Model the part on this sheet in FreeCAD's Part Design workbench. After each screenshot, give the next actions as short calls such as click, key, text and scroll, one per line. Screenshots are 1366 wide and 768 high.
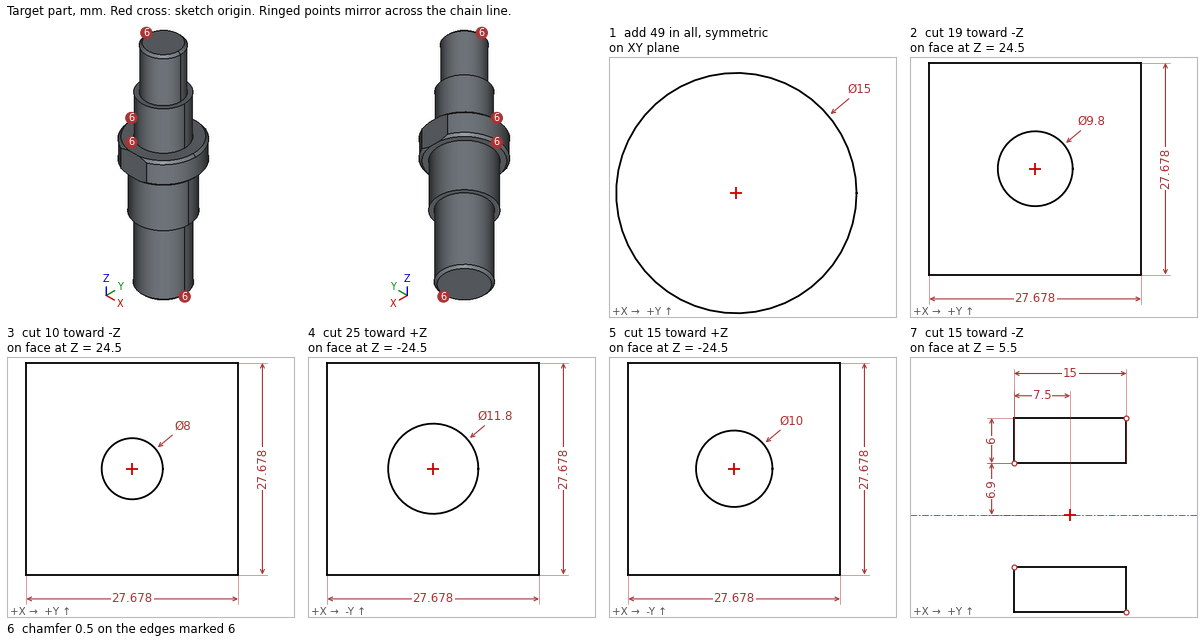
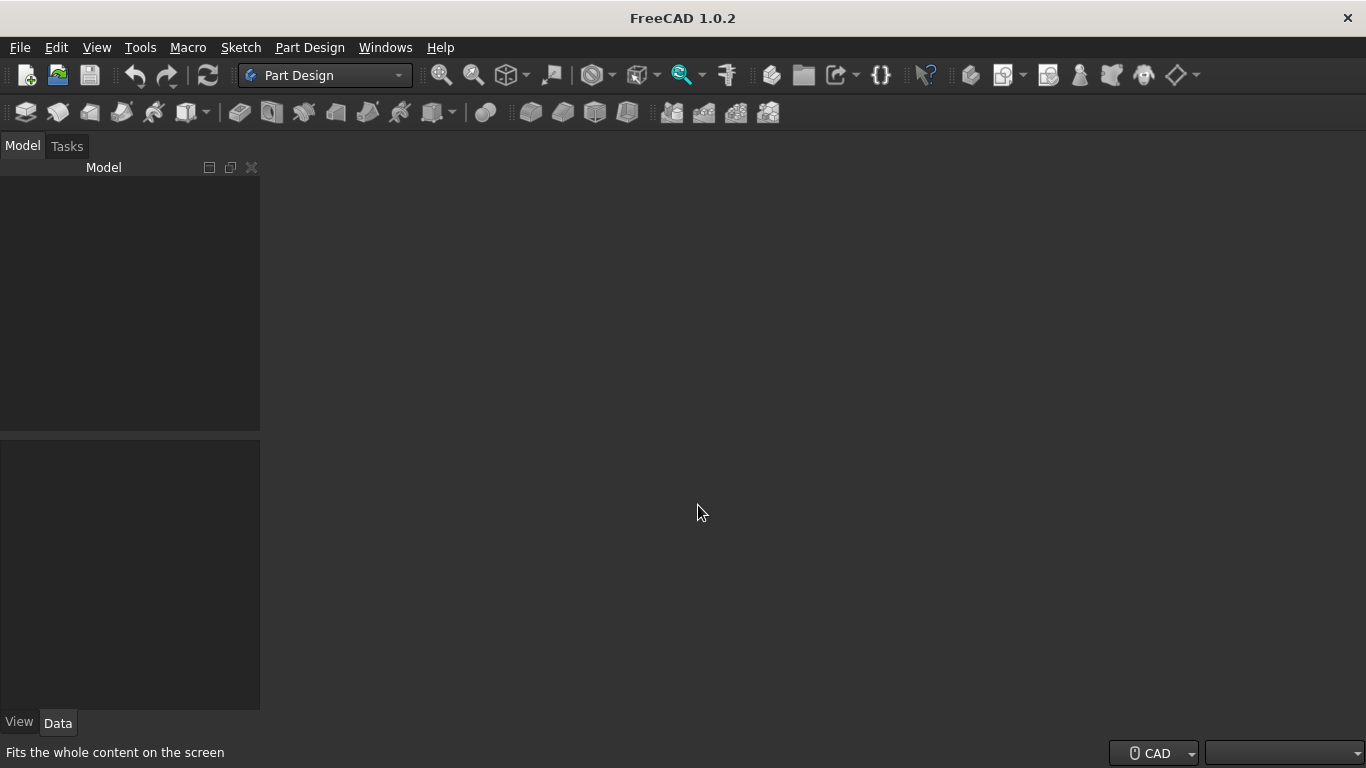
click(26, 76)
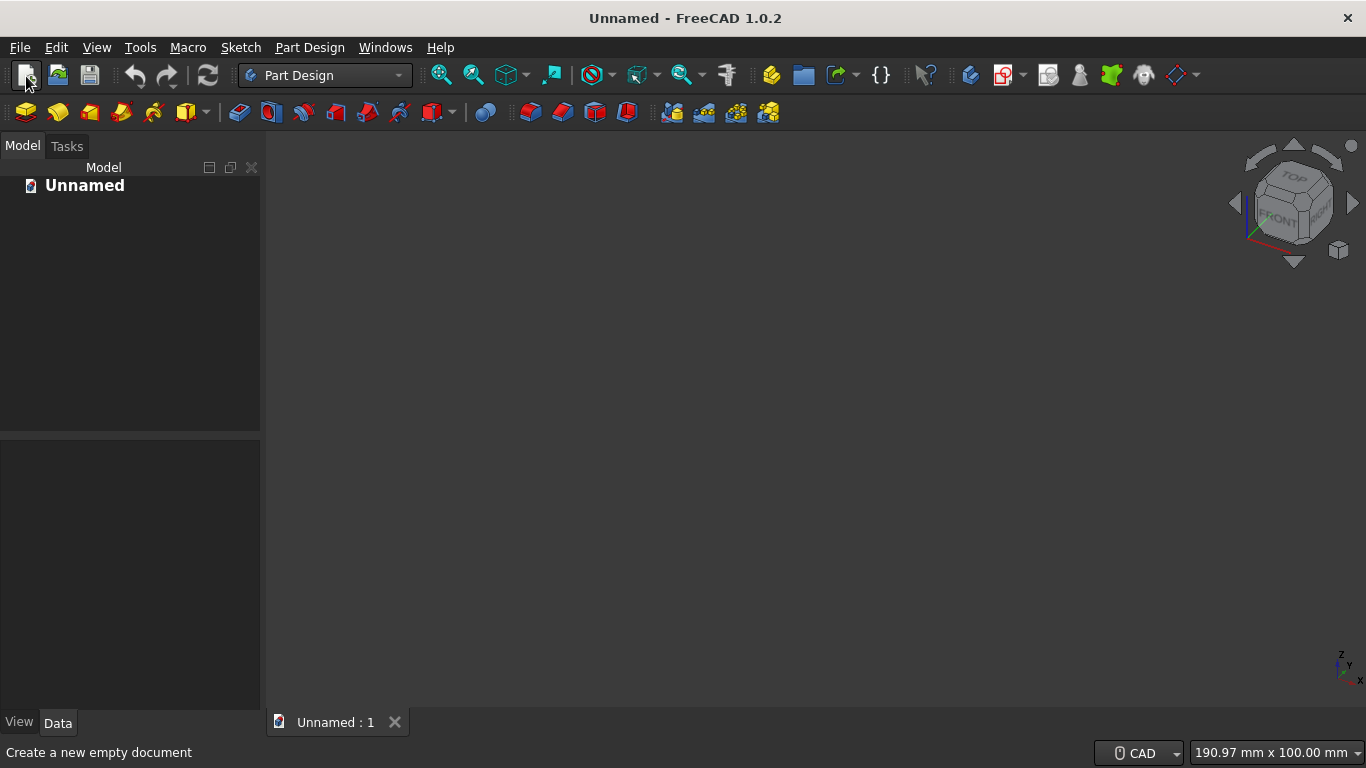
click(1004, 76)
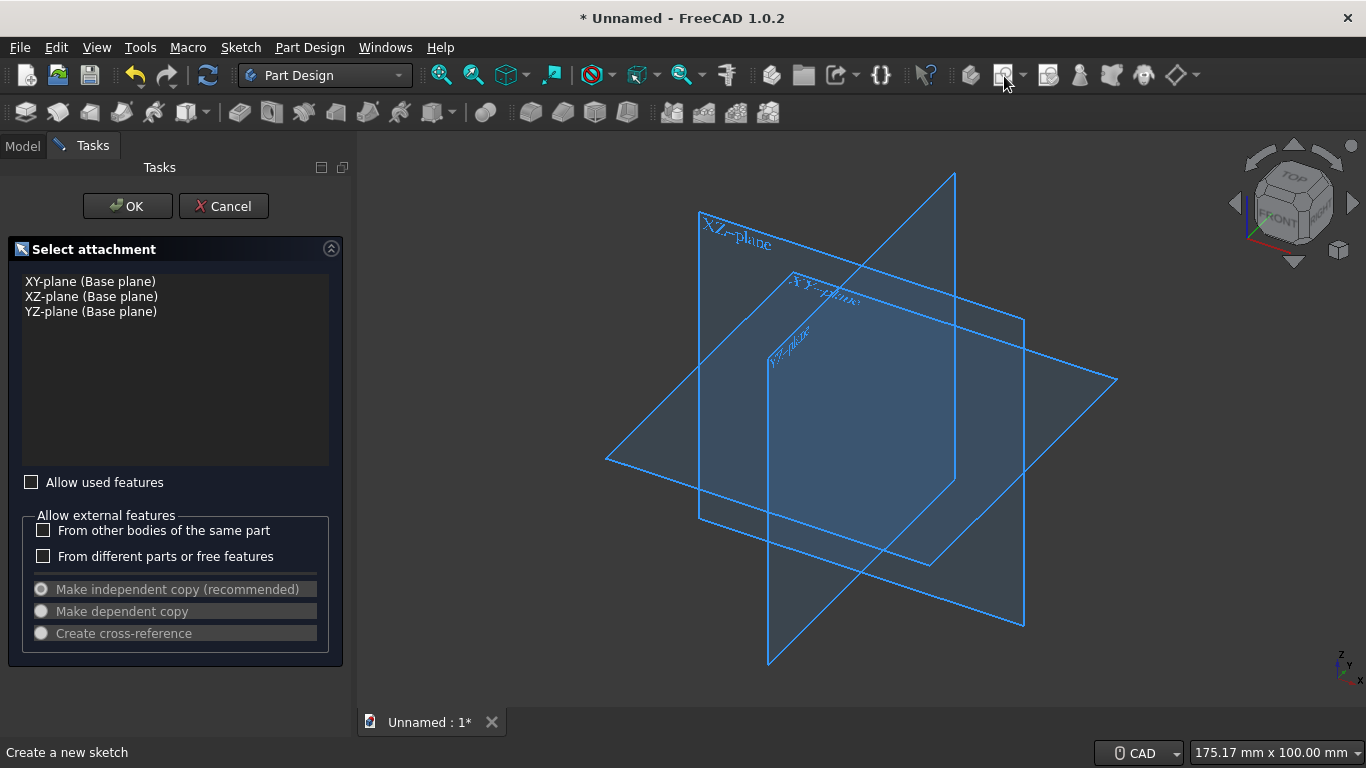
click(82, 282)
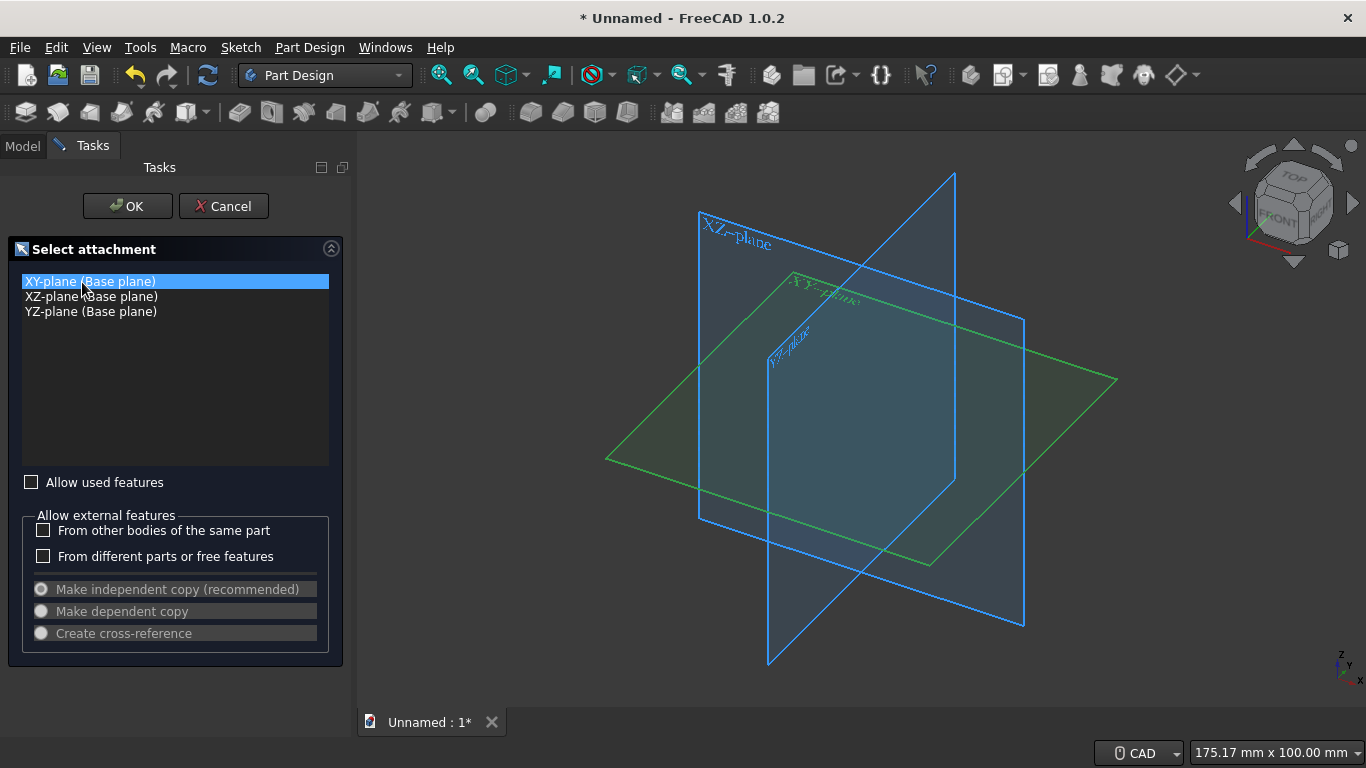
click(128, 206)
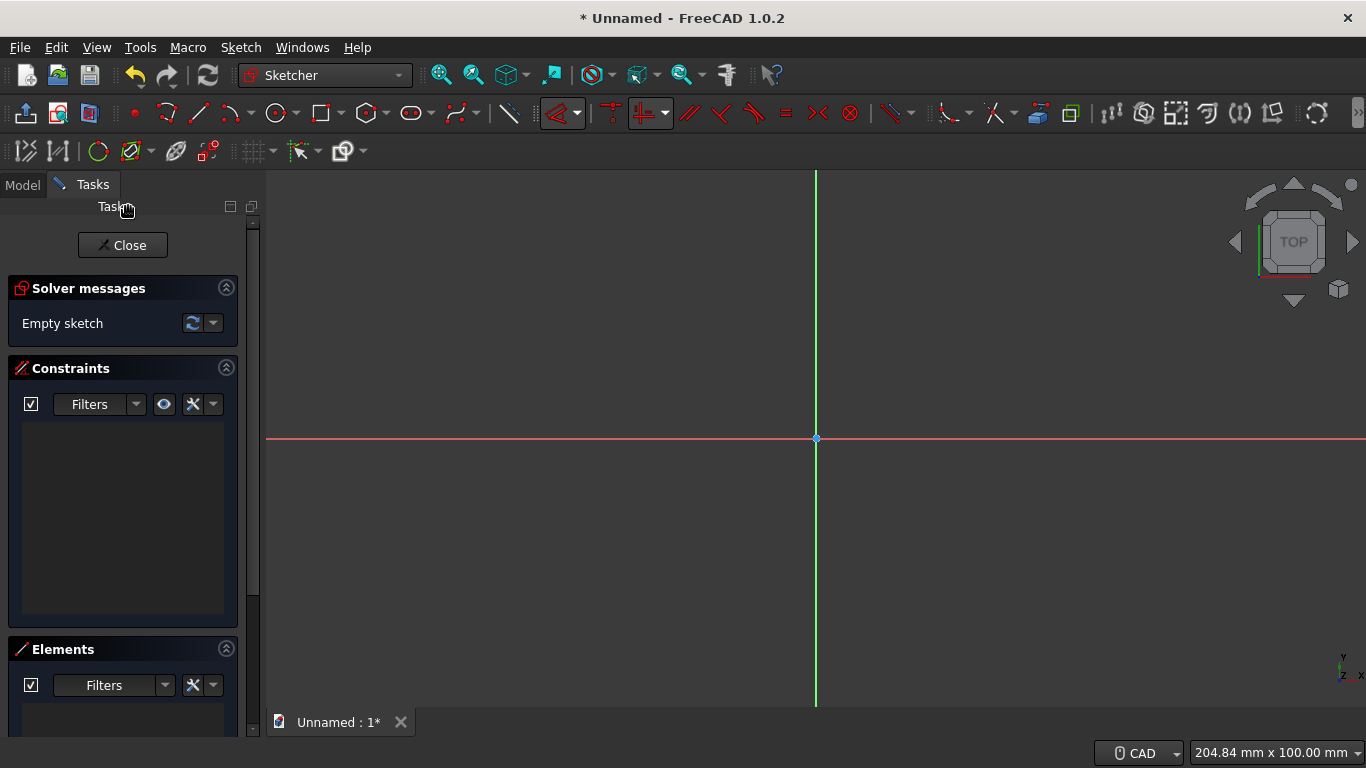
scroll(838, 438, up, 7)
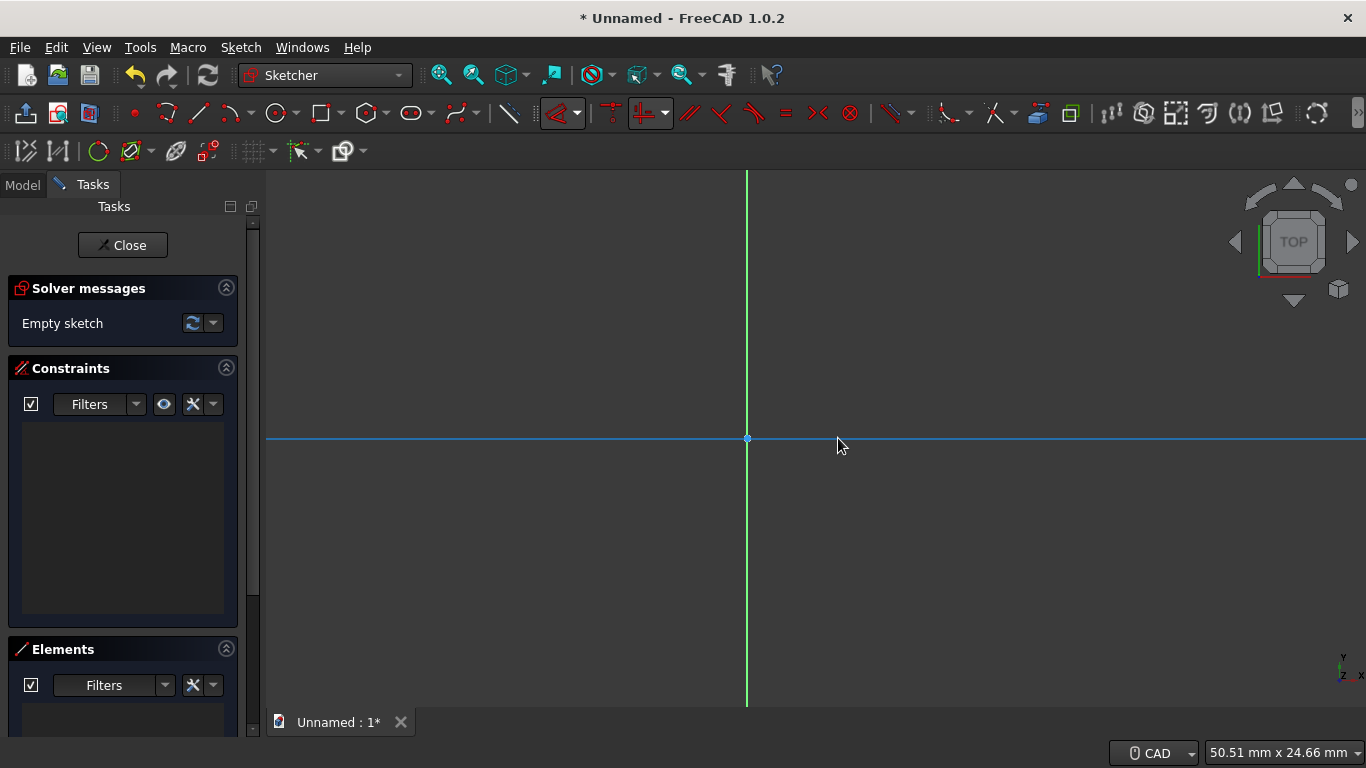
click(276, 114)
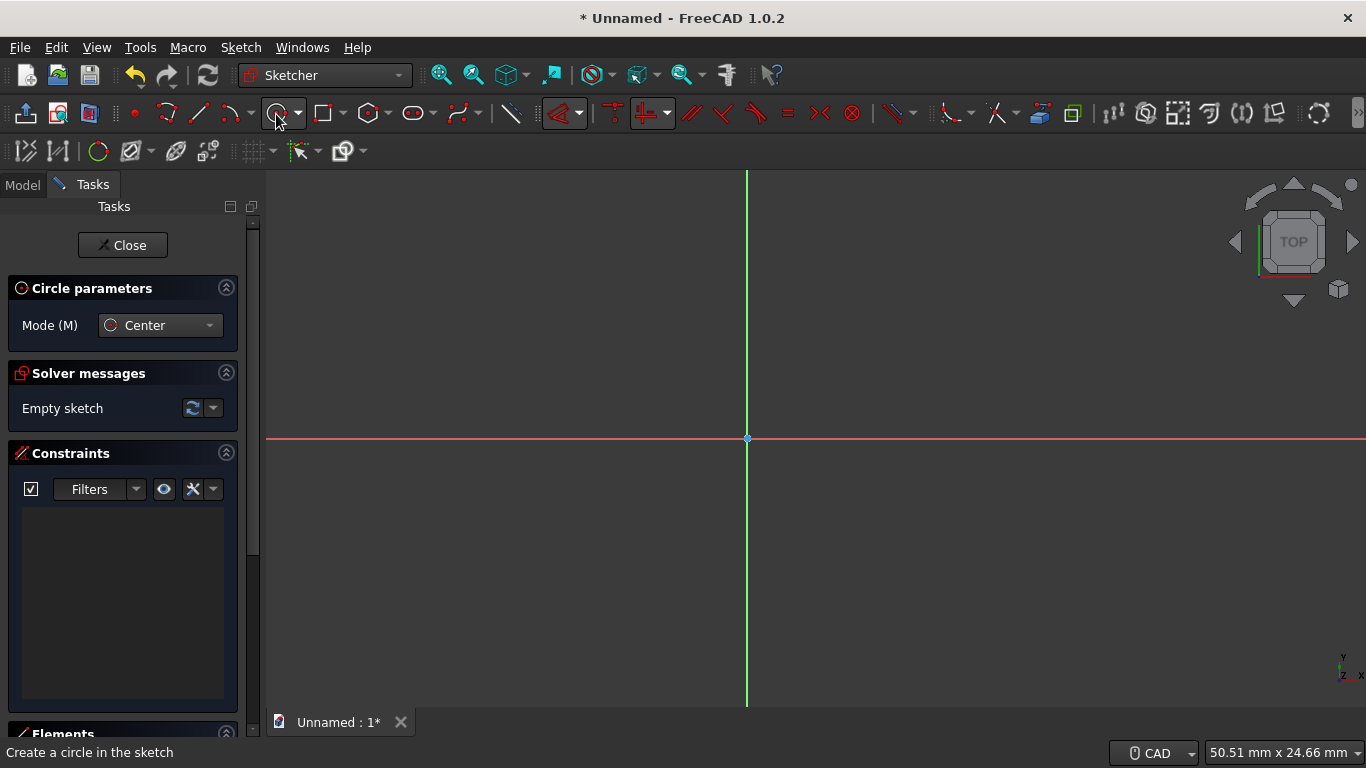
click(747, 438)
click(863, 323)
key(Escape)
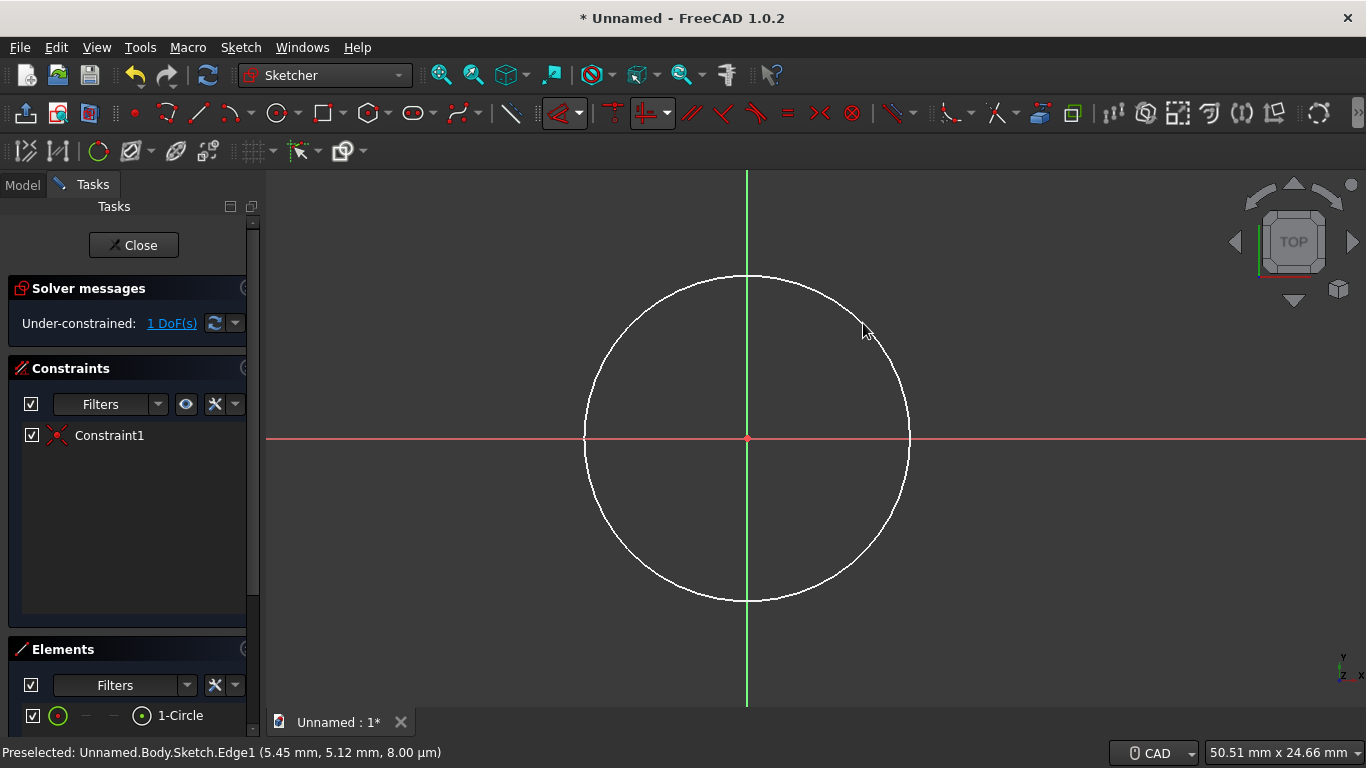
click(862, 323)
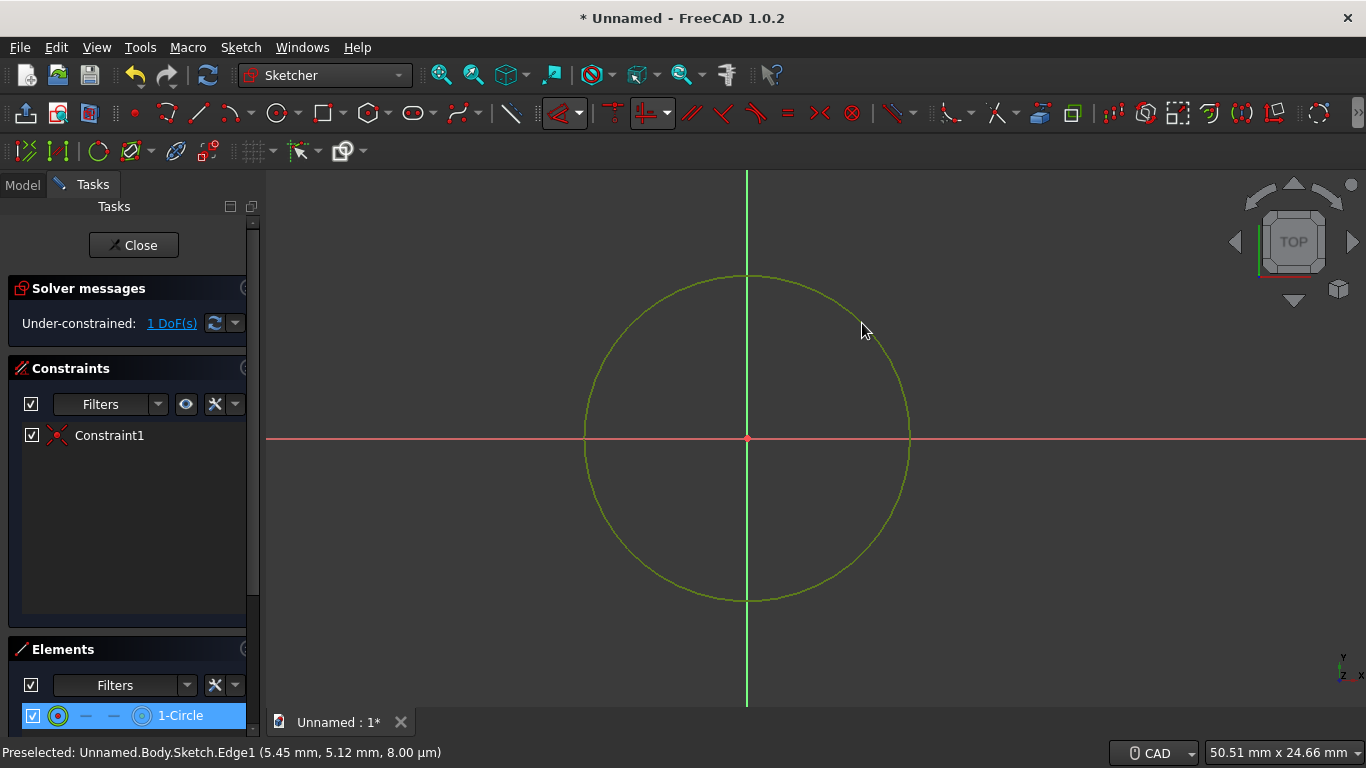
key(k)
key(o)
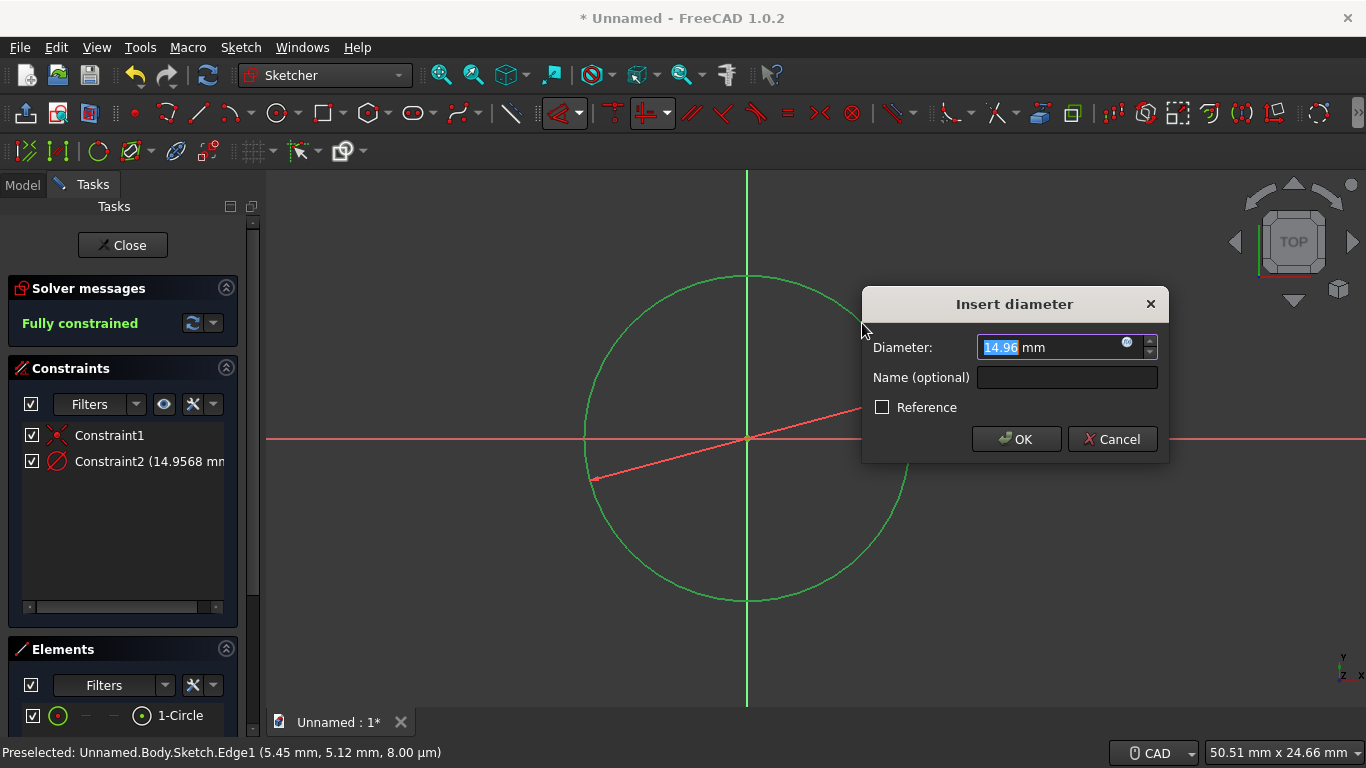
text(15)
key(Return)